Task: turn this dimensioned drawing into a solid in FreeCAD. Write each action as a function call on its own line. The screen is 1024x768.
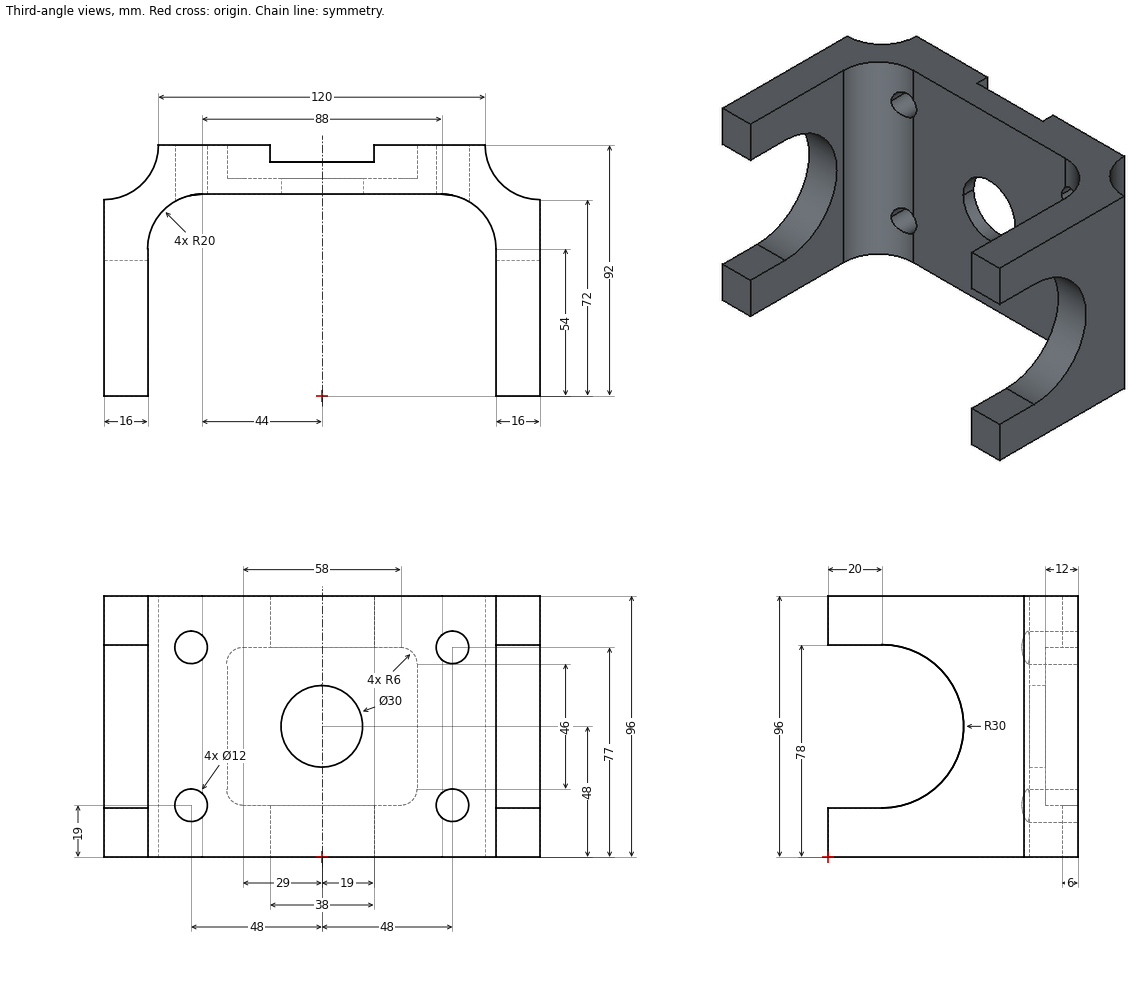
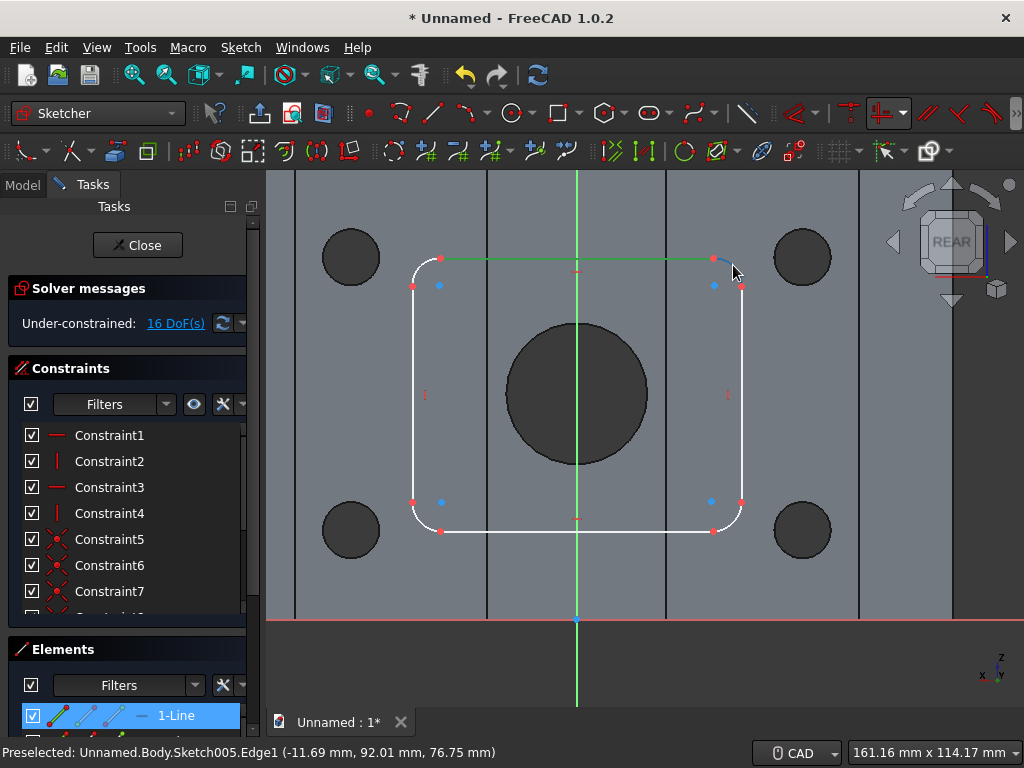
click(428, 261)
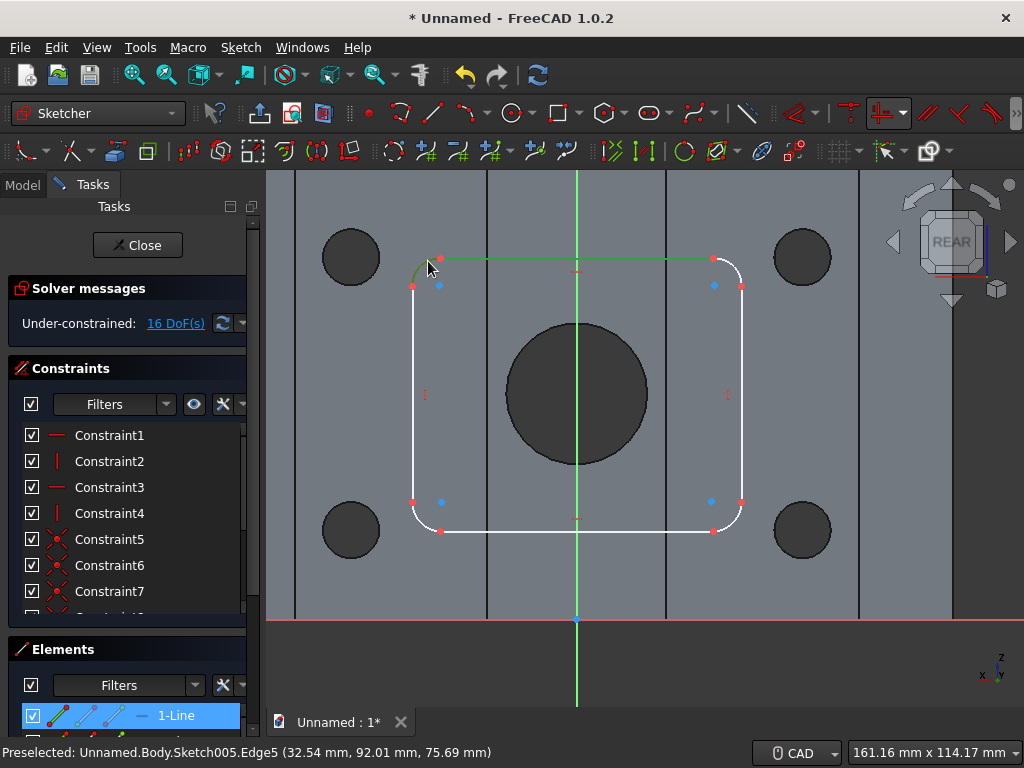
click(992, 114)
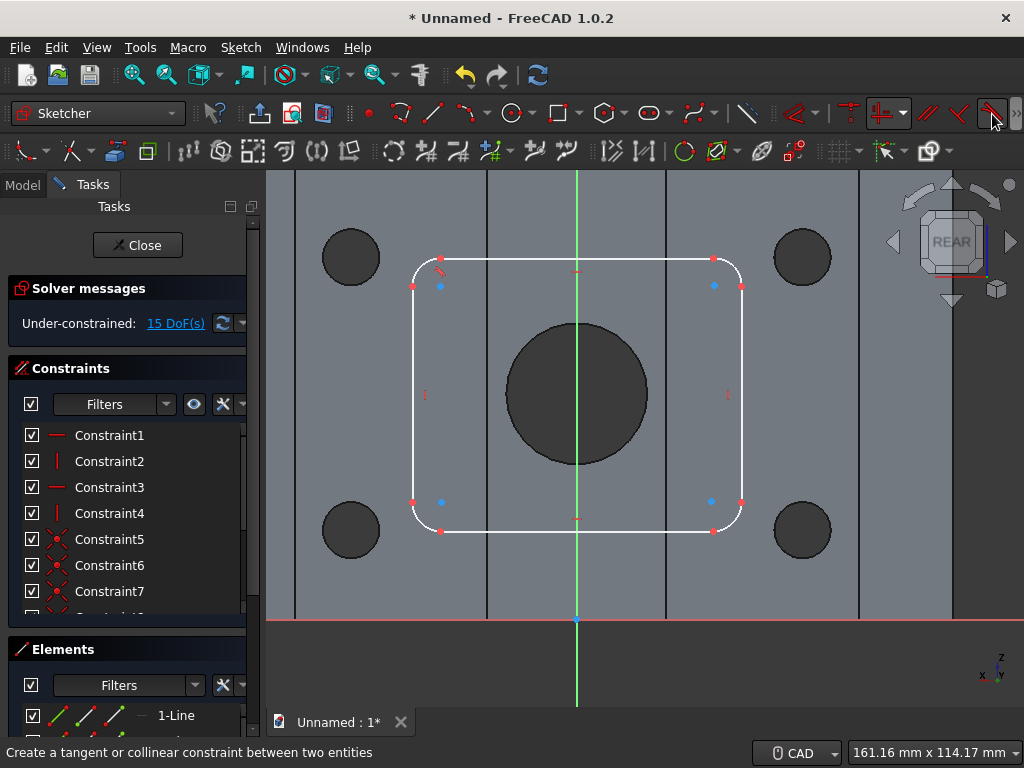
click(632, 259)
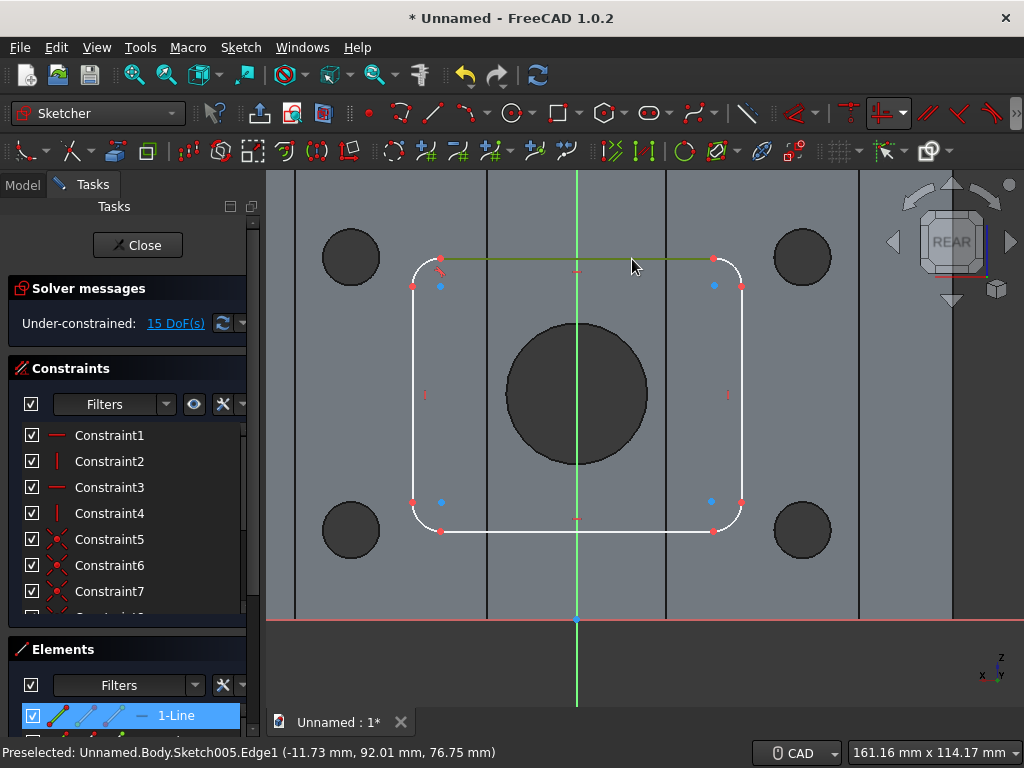
click(739, 274)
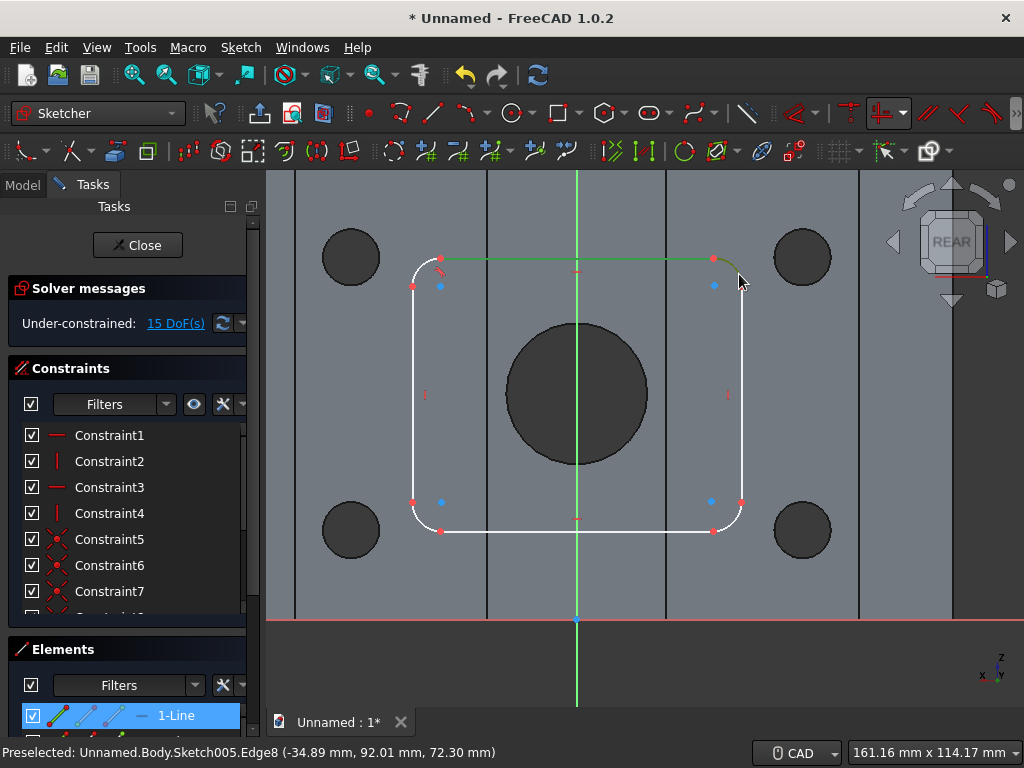
click(992, 114)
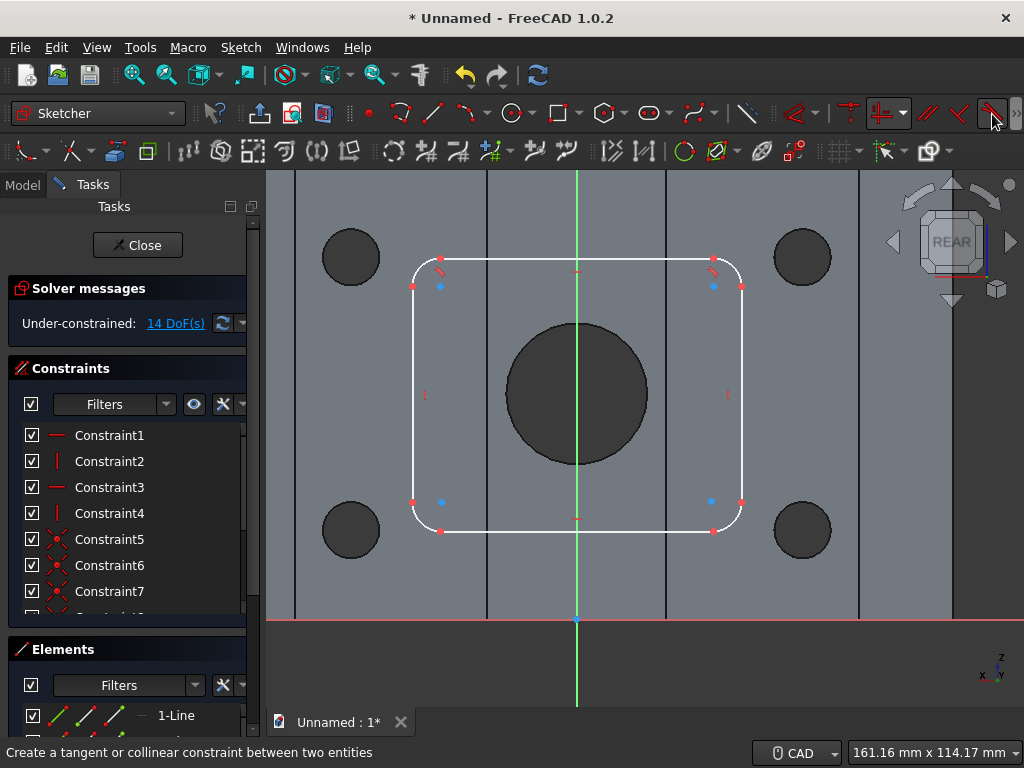
click(413, 351)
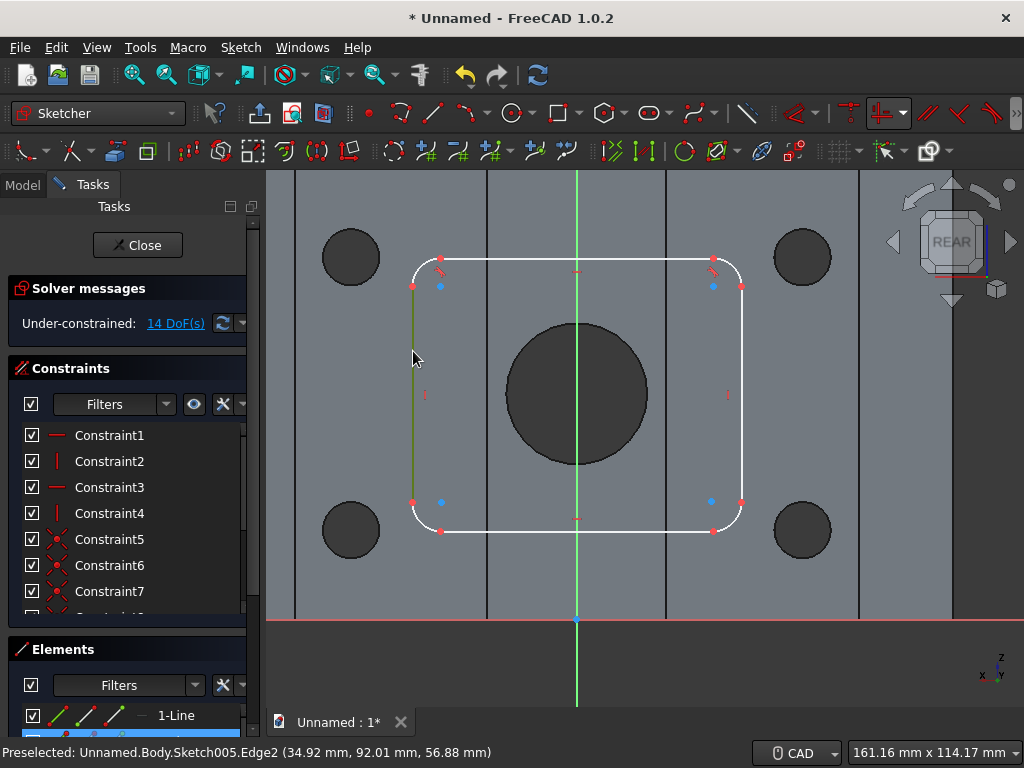
click(428, 262)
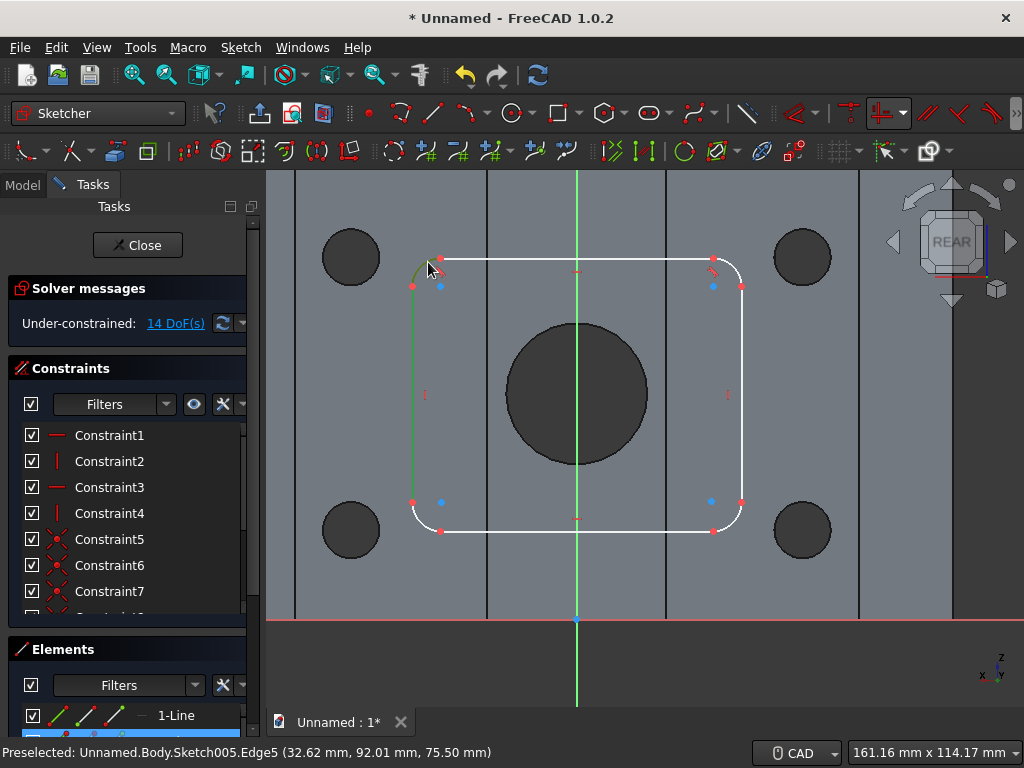
click(992, 114)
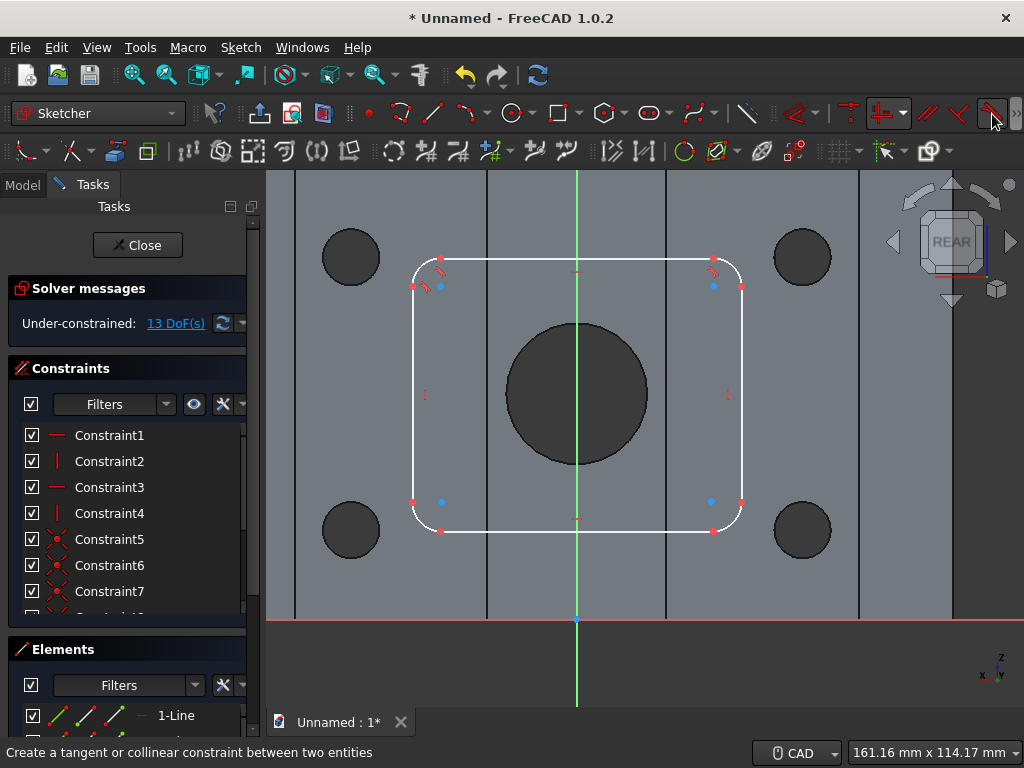
click(413, 351)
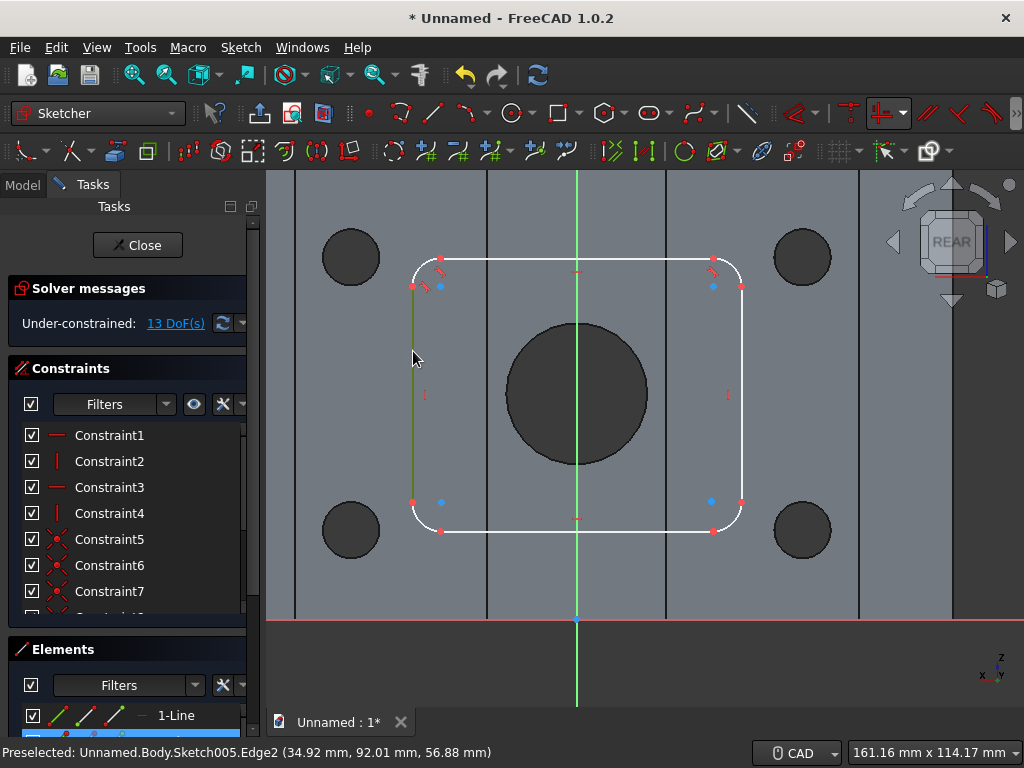
click(416, 515)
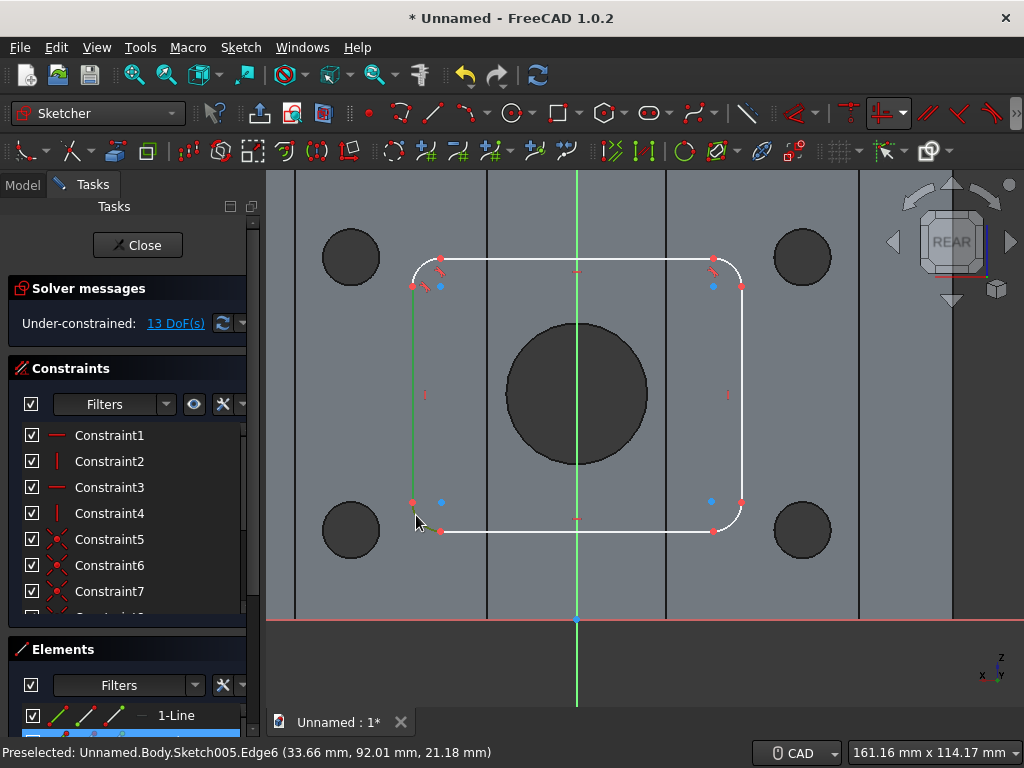
click(992, 114)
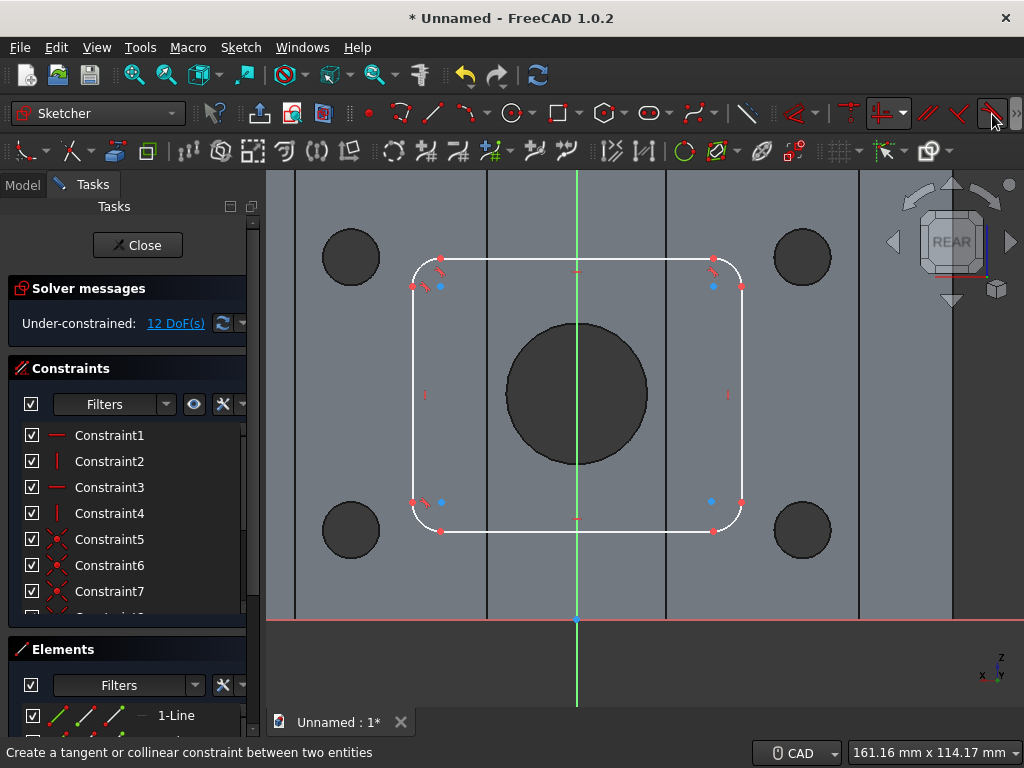
click(522, 532)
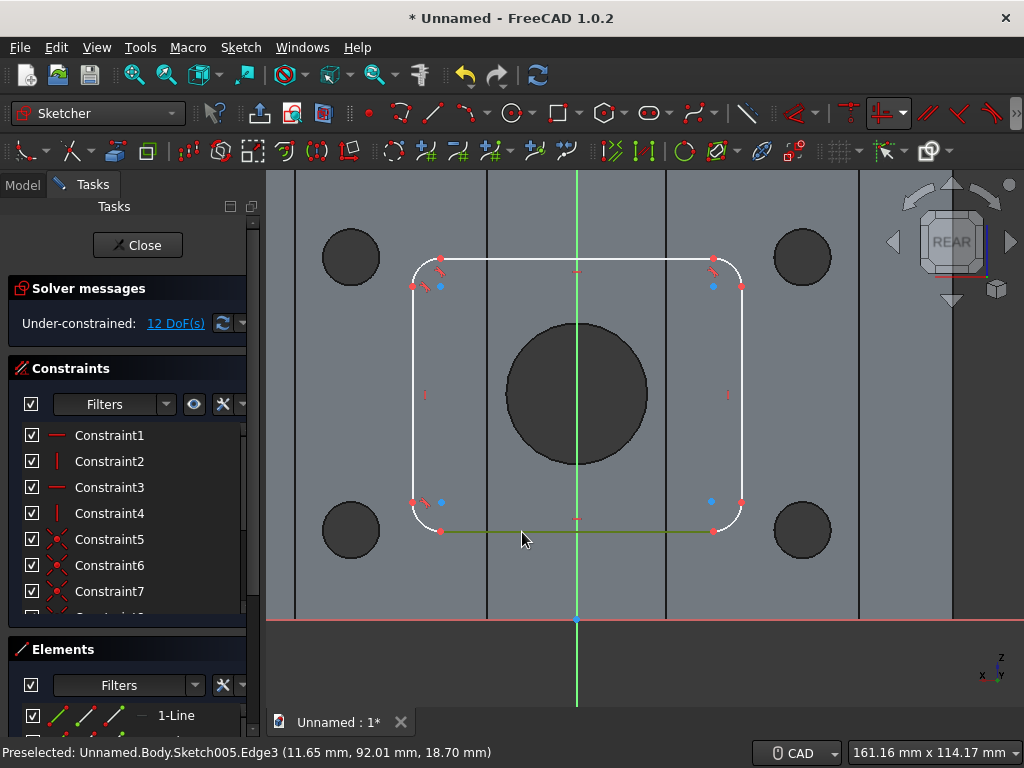
click(416, 515)